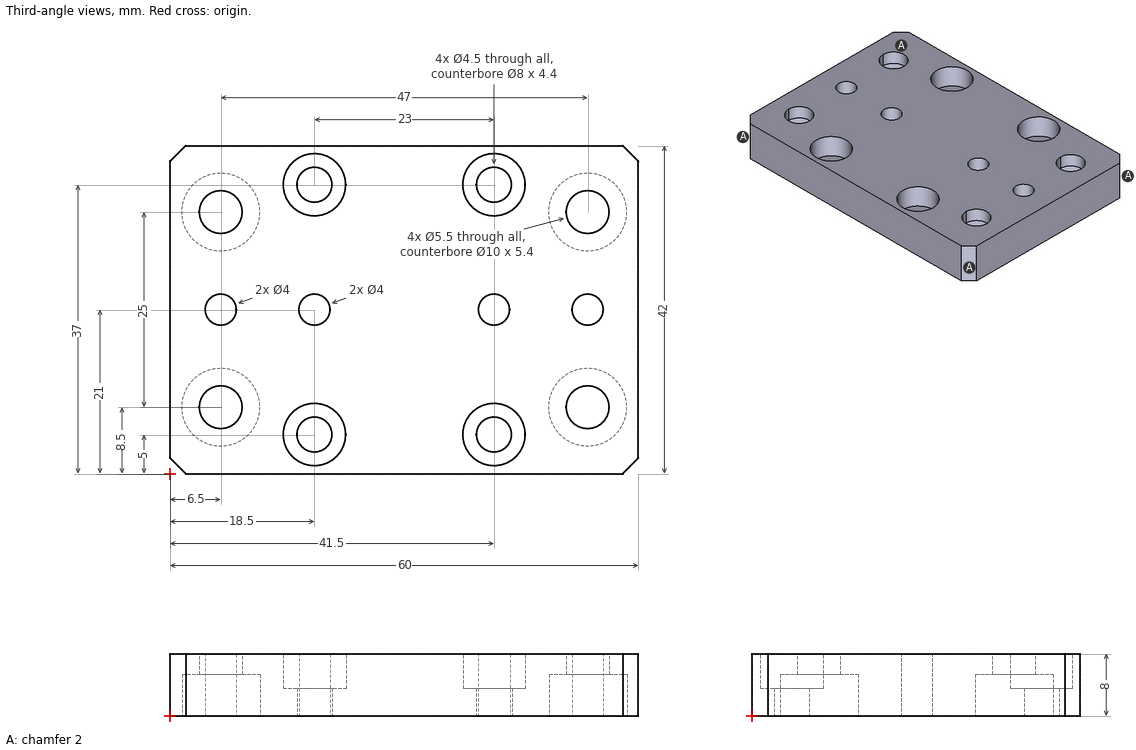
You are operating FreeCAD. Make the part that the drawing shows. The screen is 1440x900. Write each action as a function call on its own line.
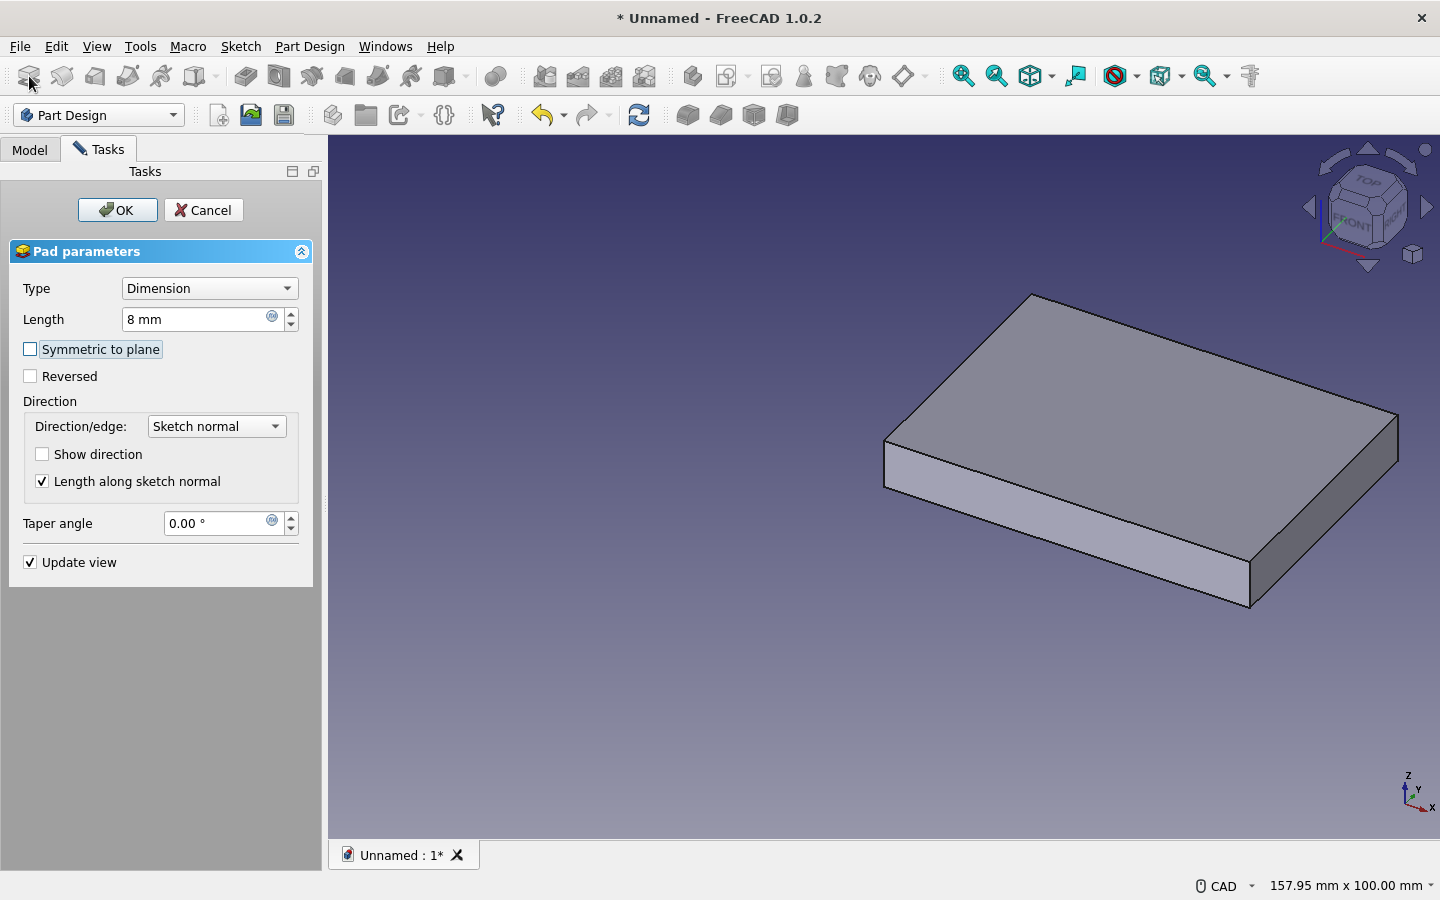
click(118, 210)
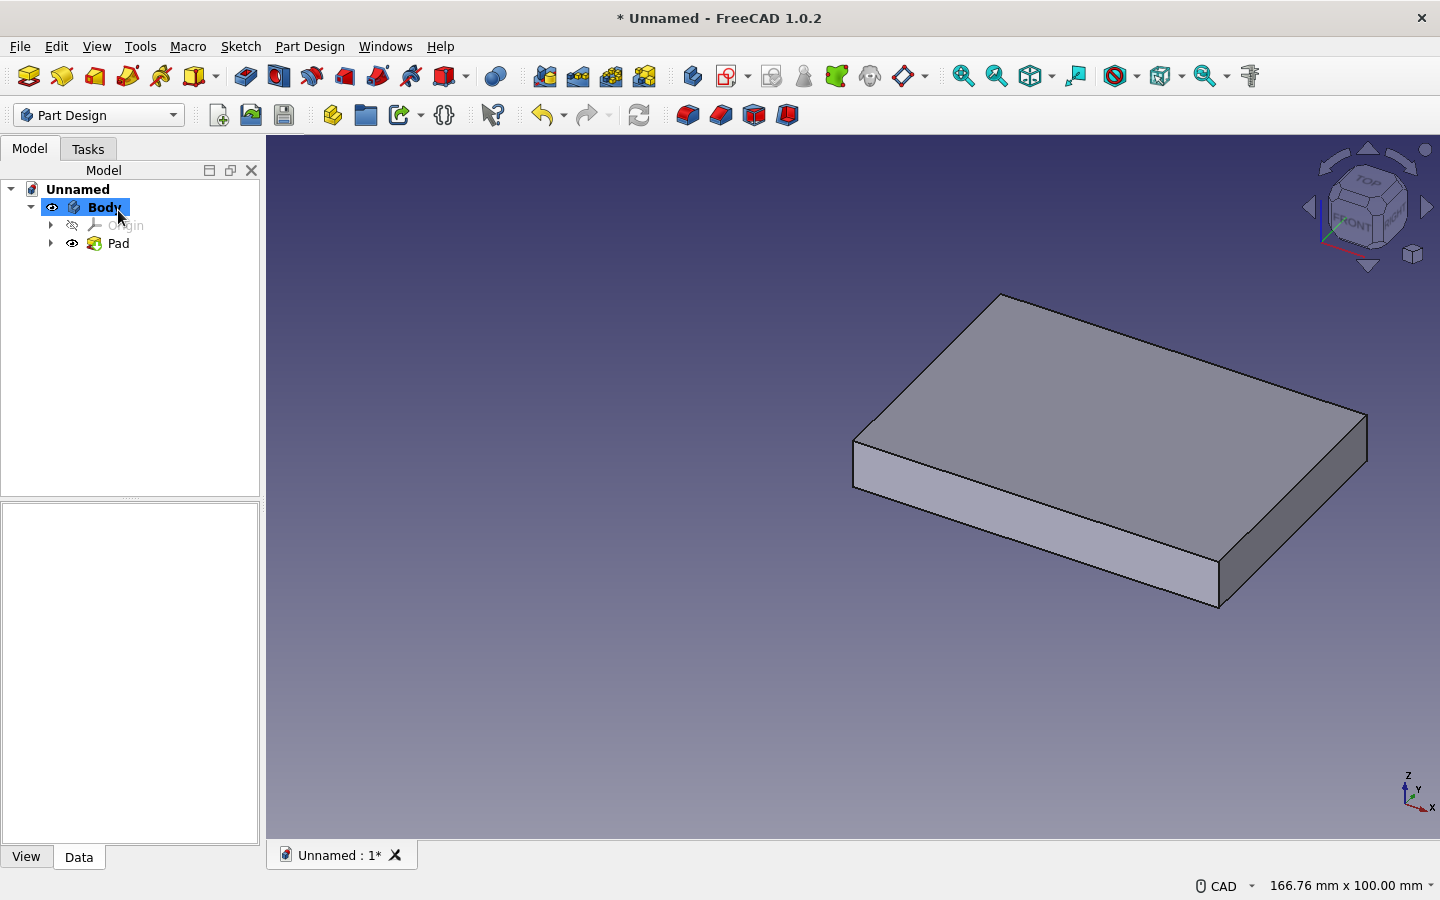
click(964, 76)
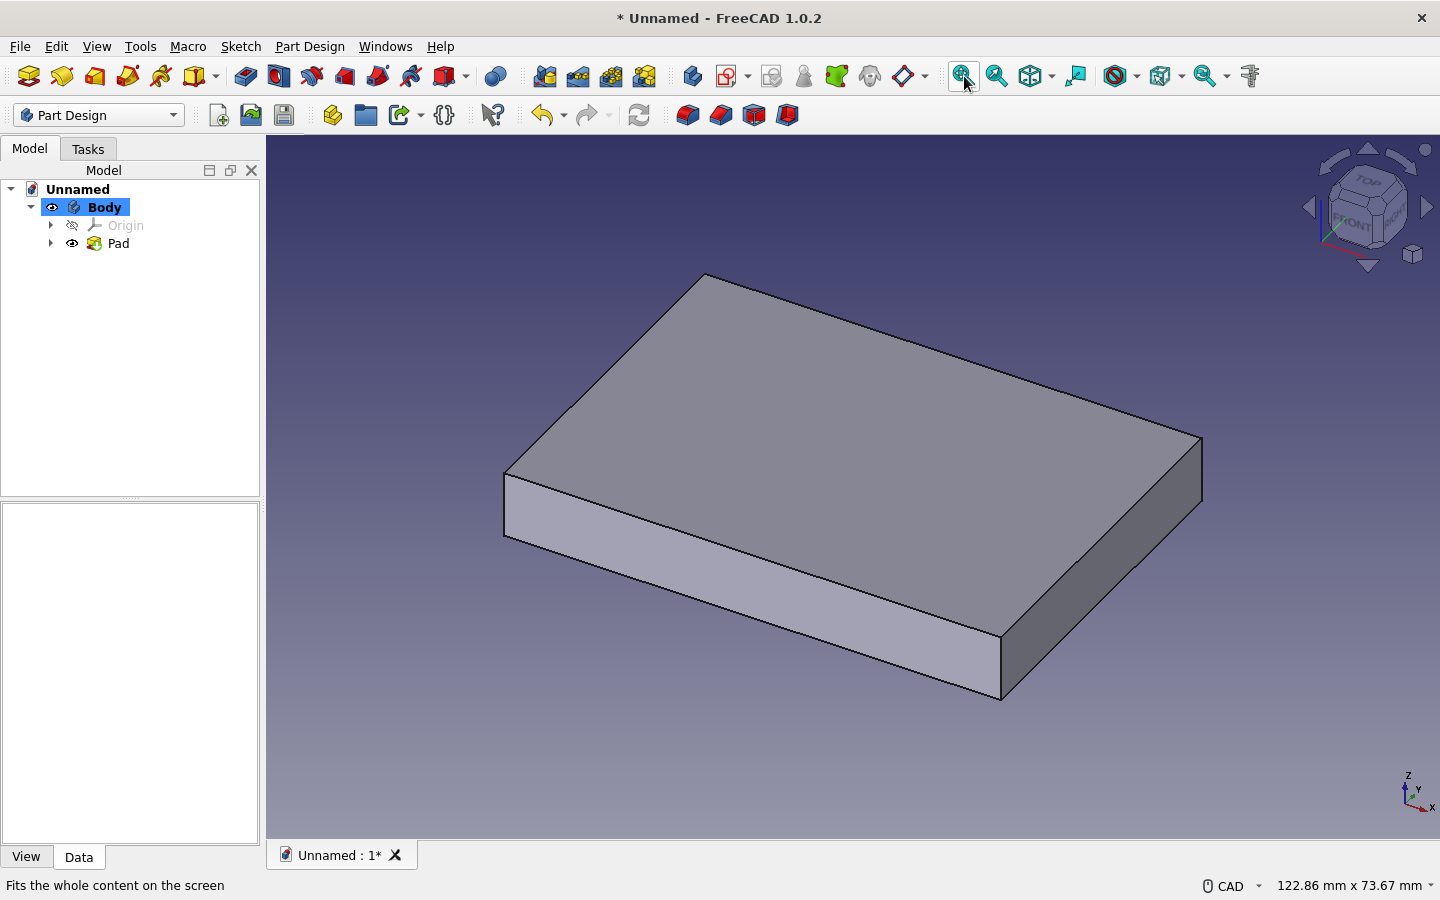
click(924, 478)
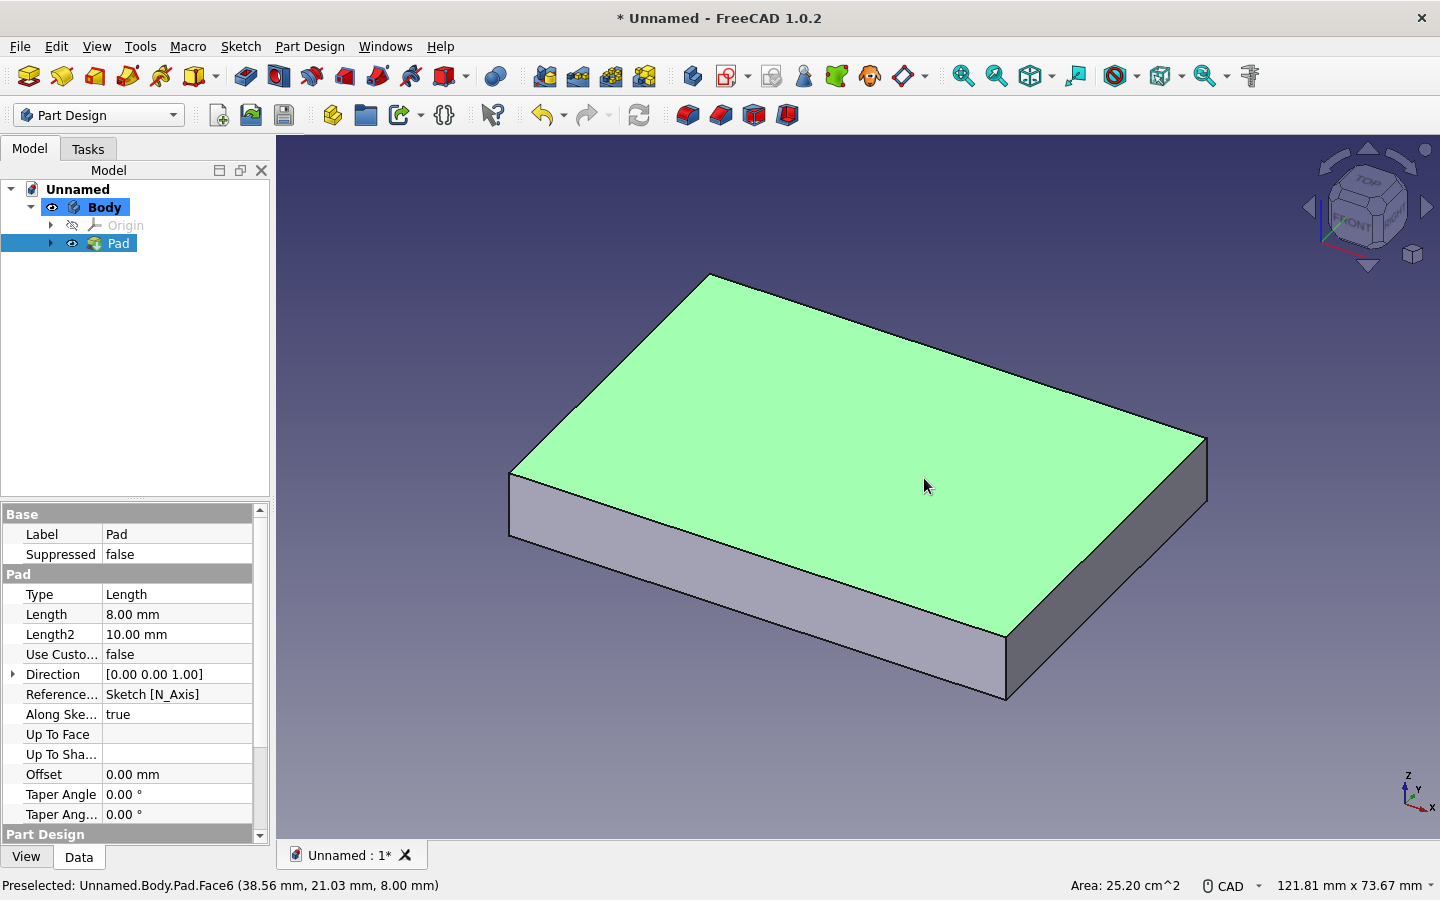
click(726, 76)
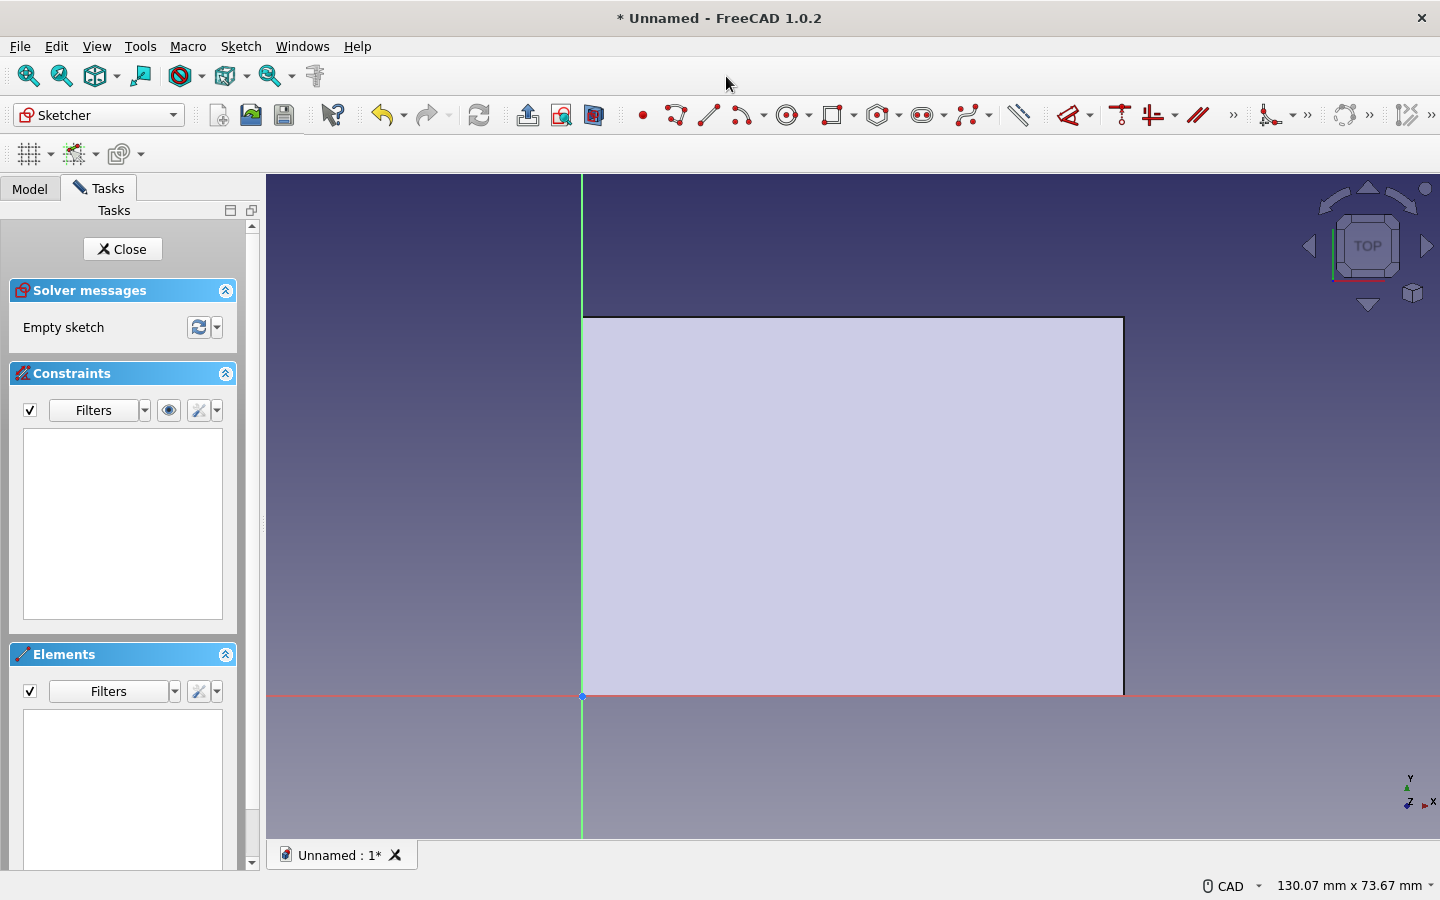
click(786, 116)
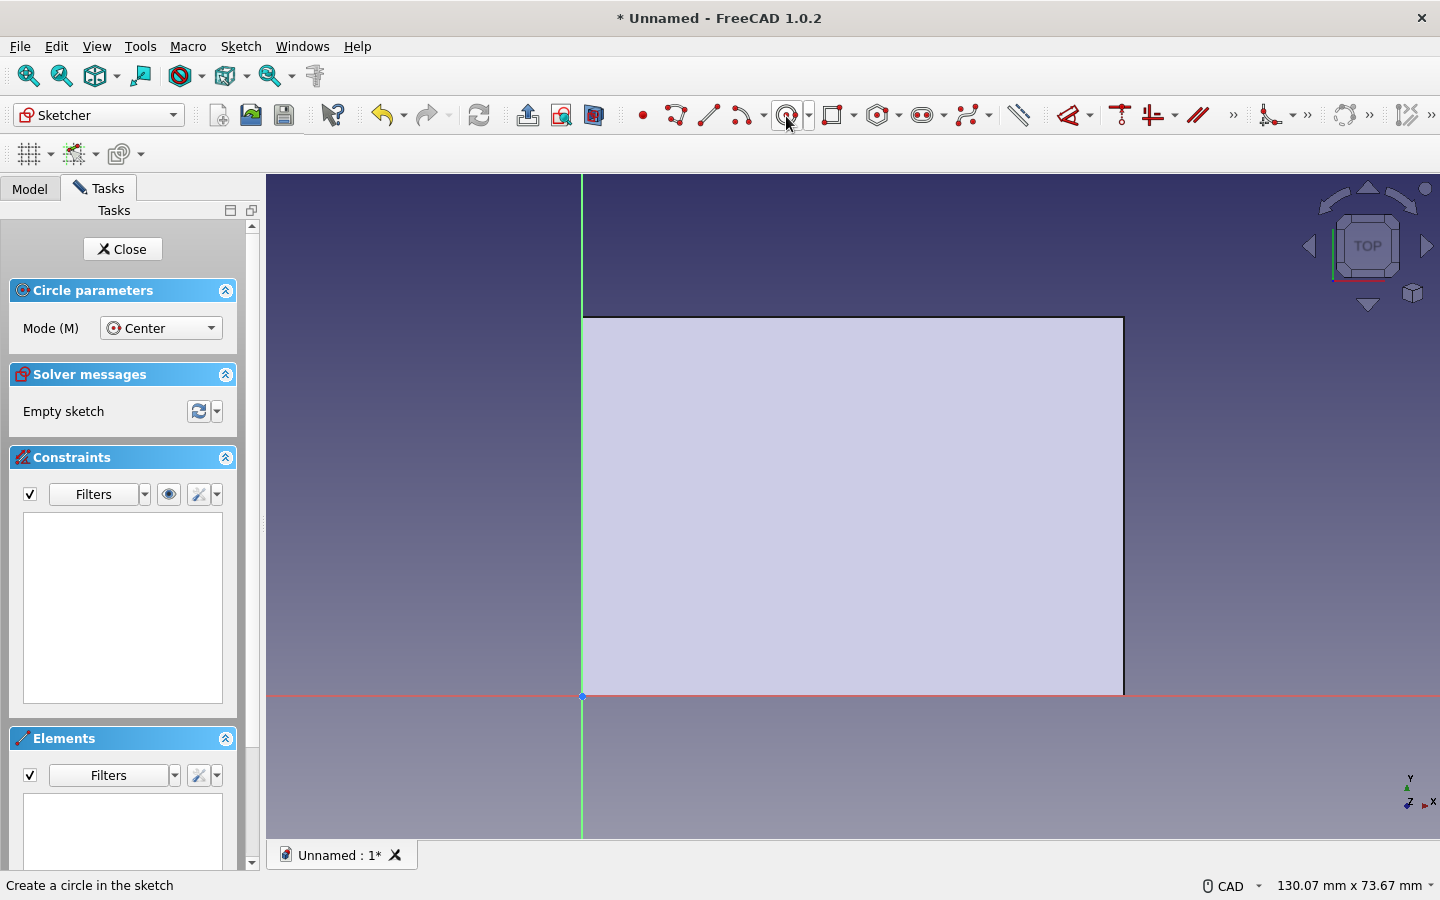
click(957, 362)
click(971, 348)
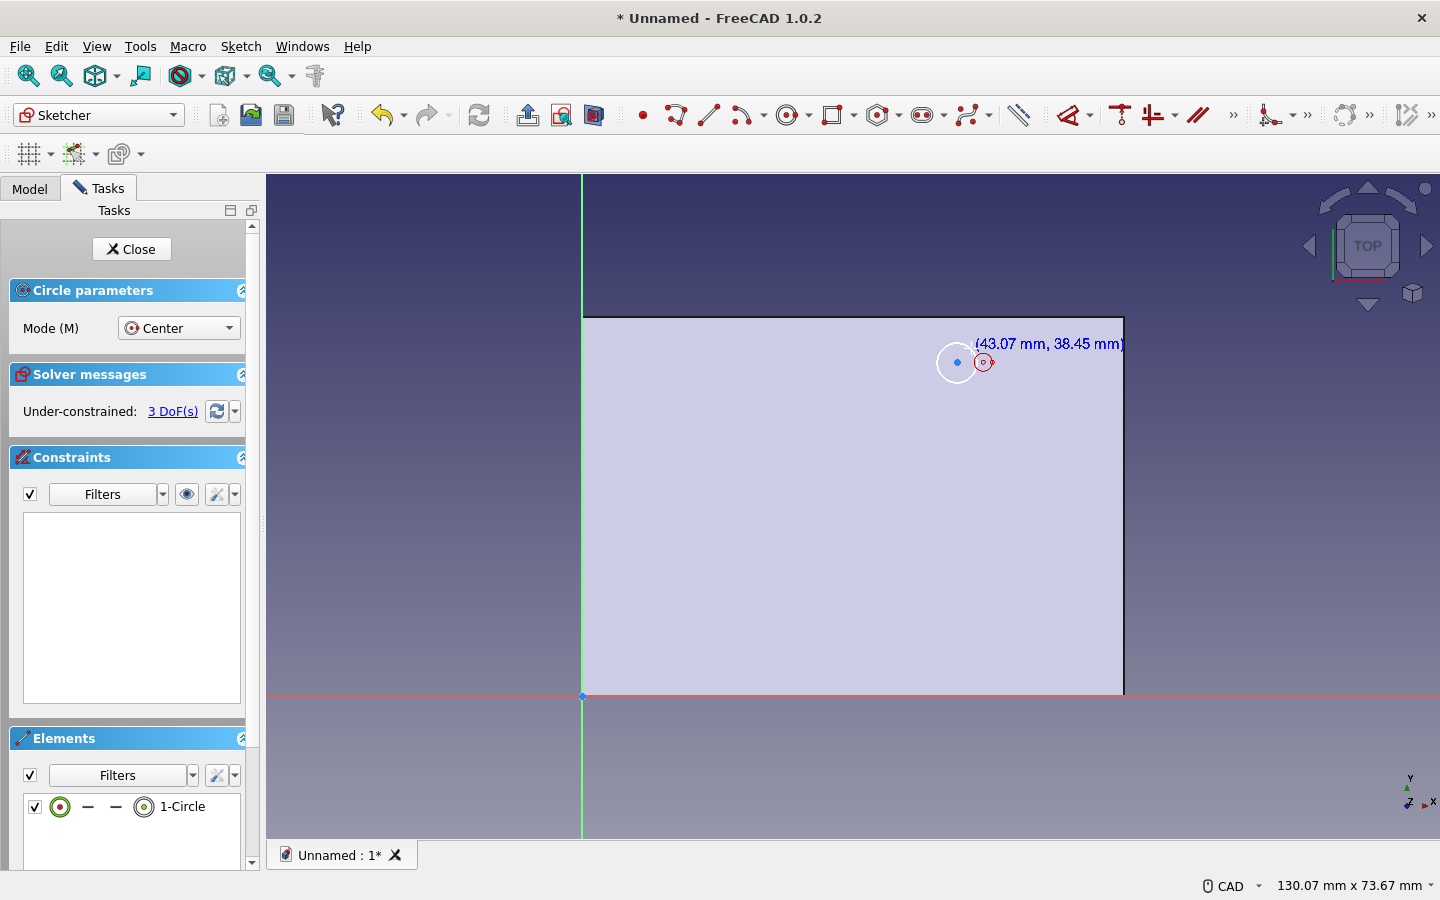
click(749, 362)
click(764, 348)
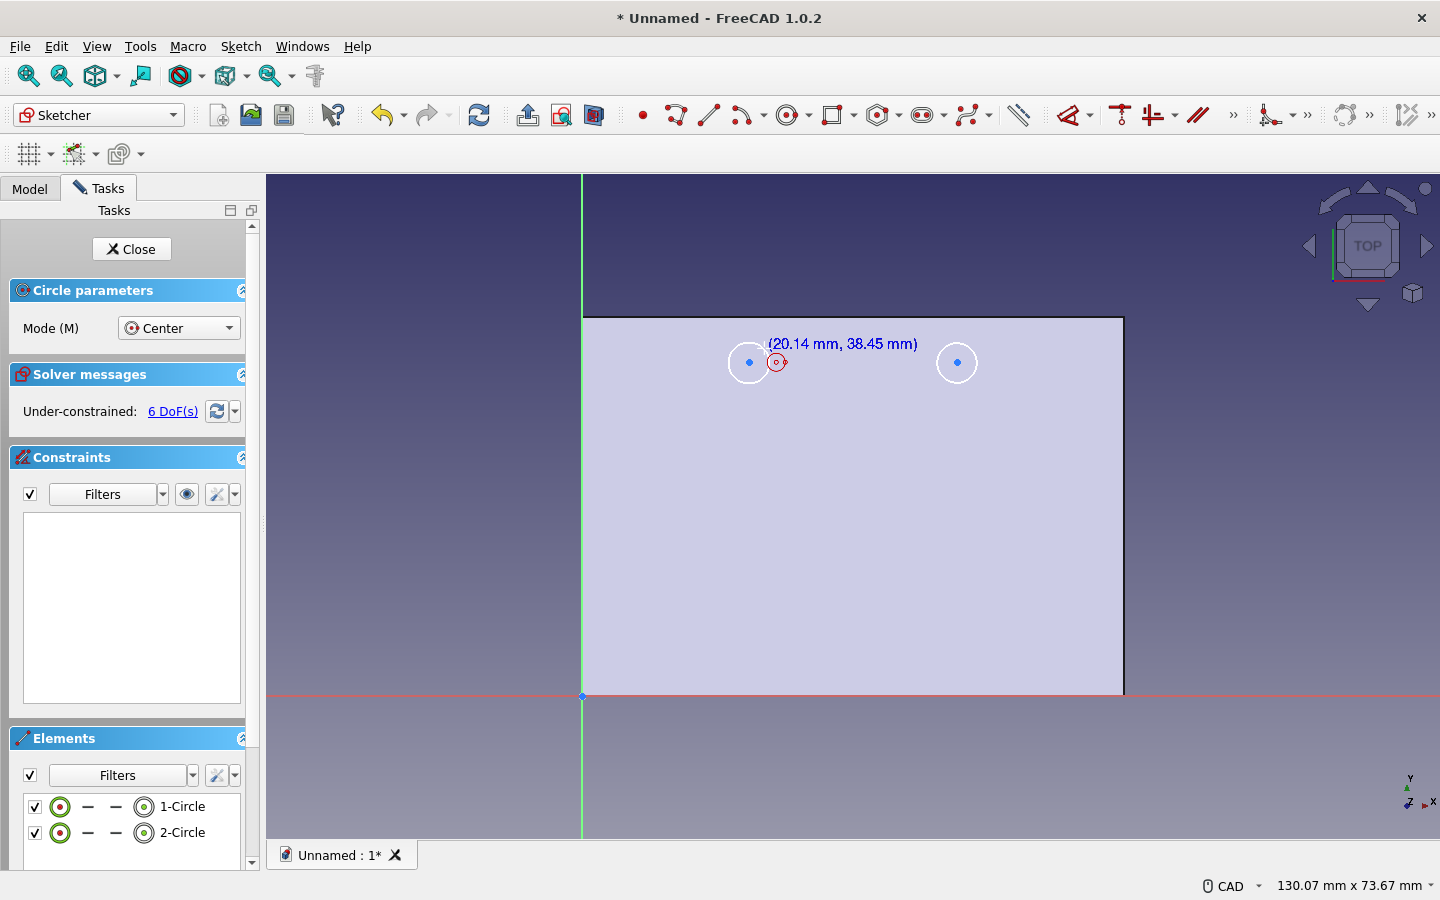
click(749, 651)
click(764, 637)